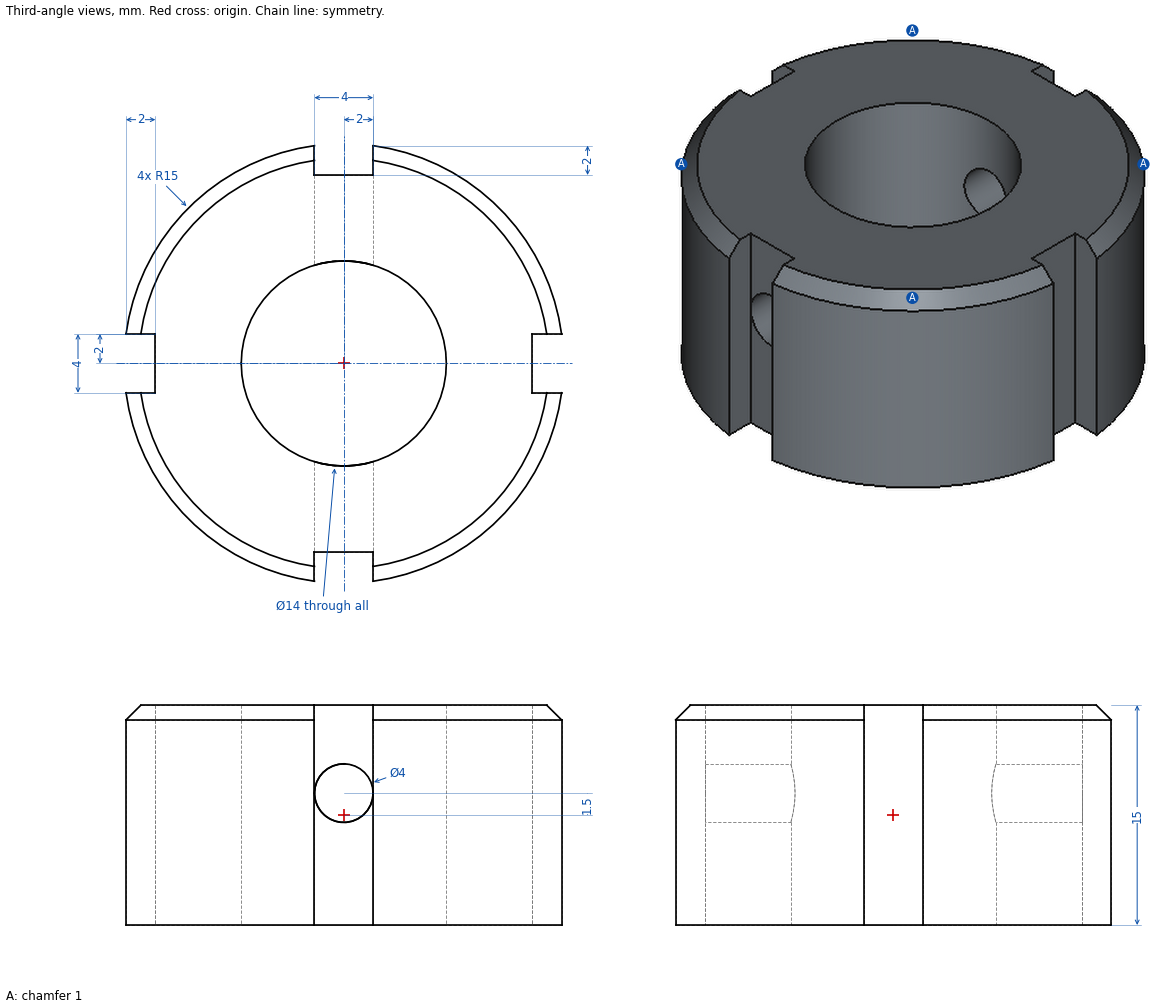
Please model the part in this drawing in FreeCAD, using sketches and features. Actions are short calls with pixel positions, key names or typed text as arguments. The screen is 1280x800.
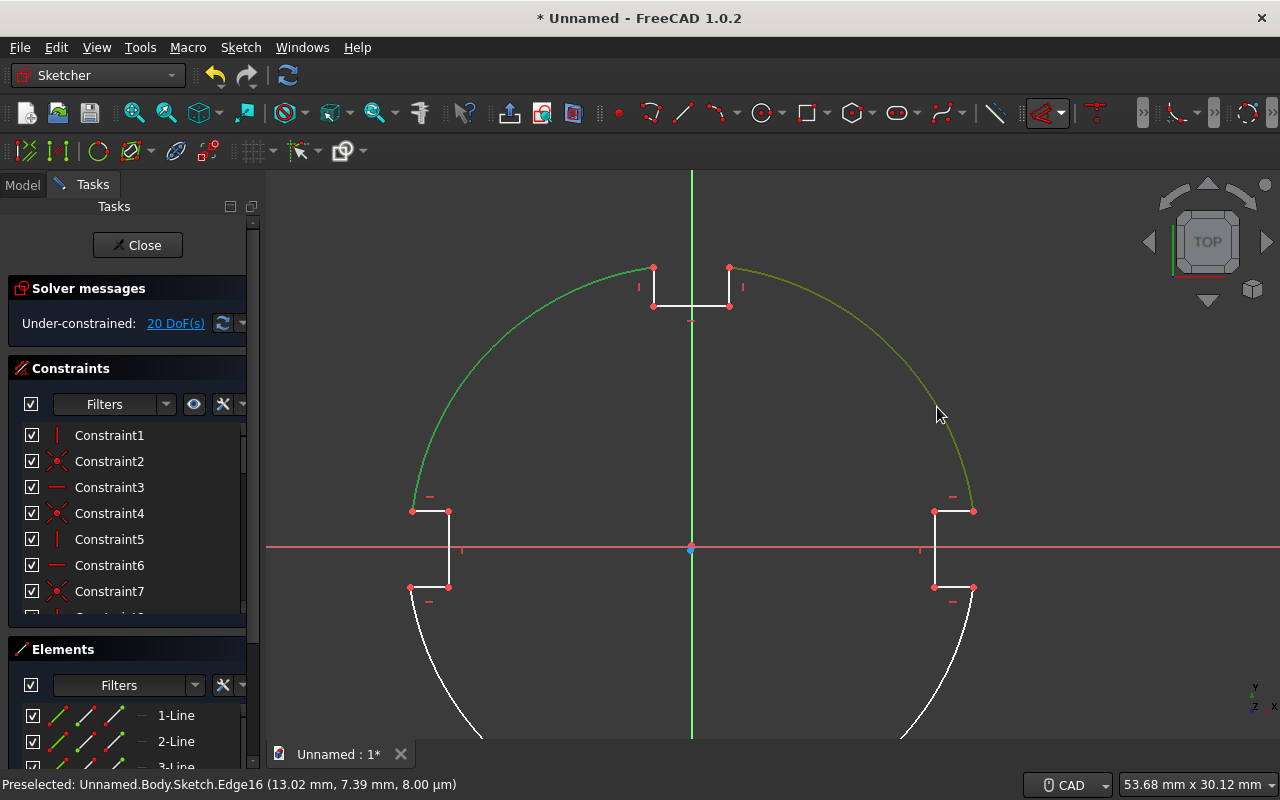
key(c)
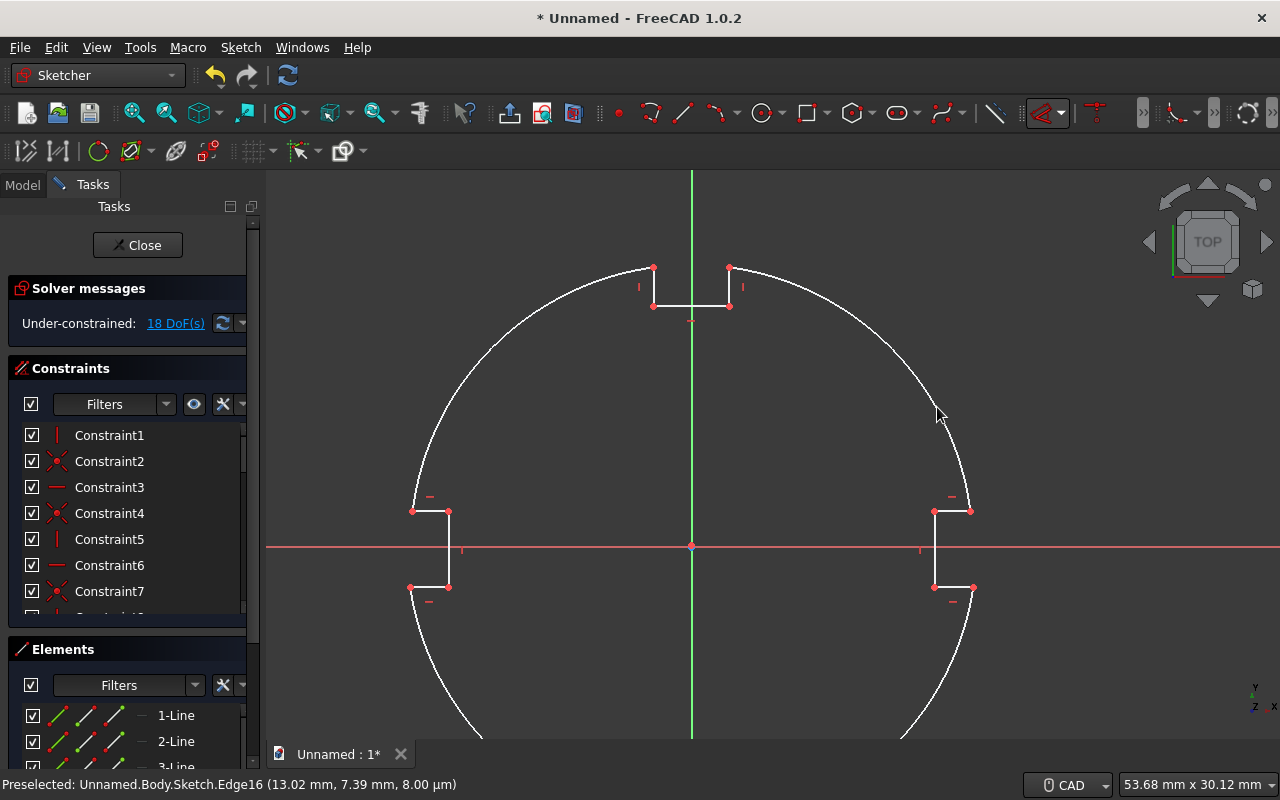
drag(682, 536, 702, 557)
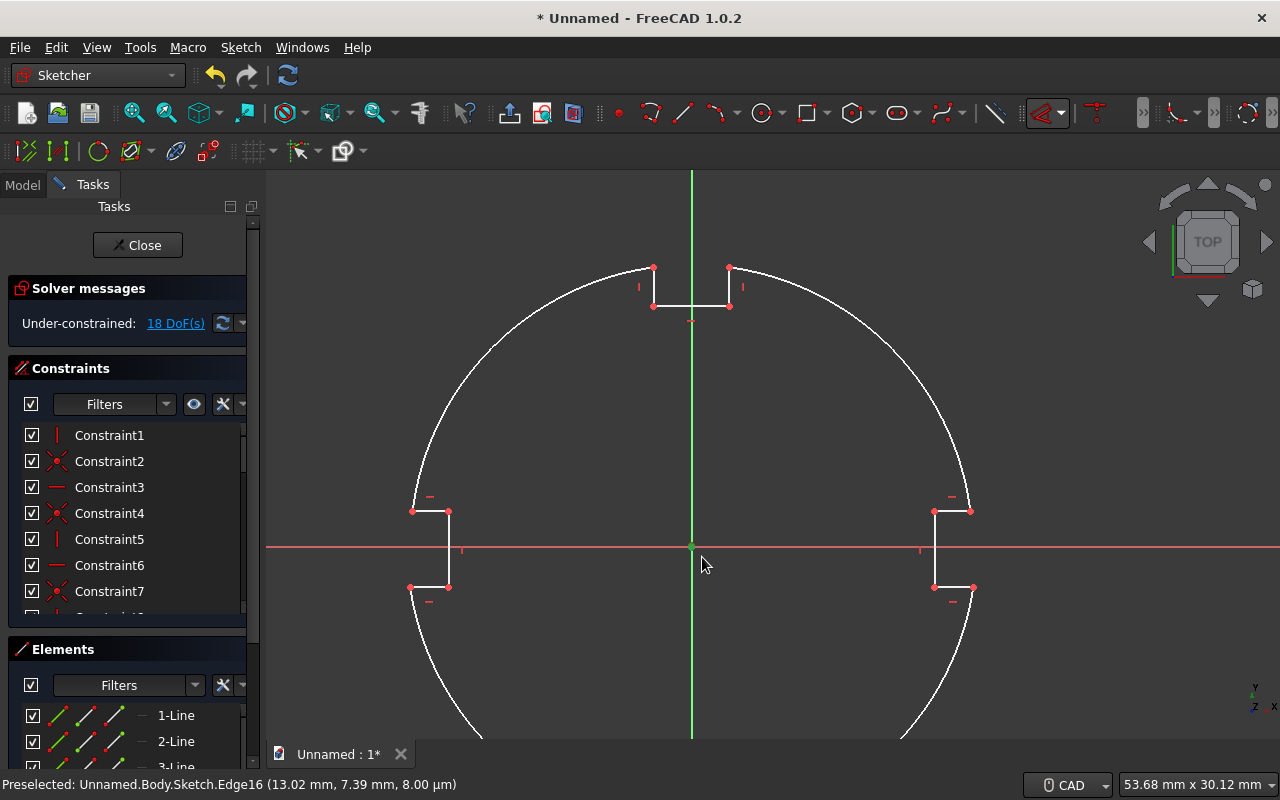
key(c)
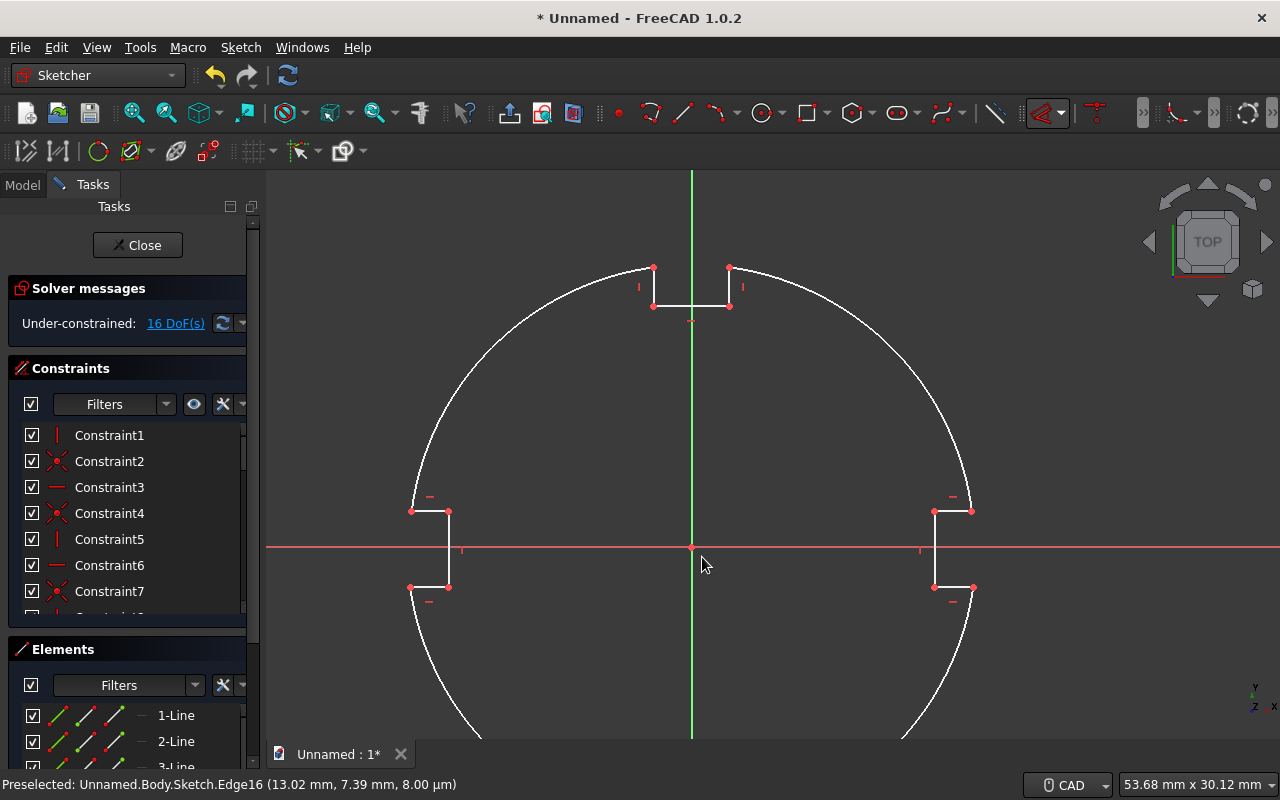
click(550, 303)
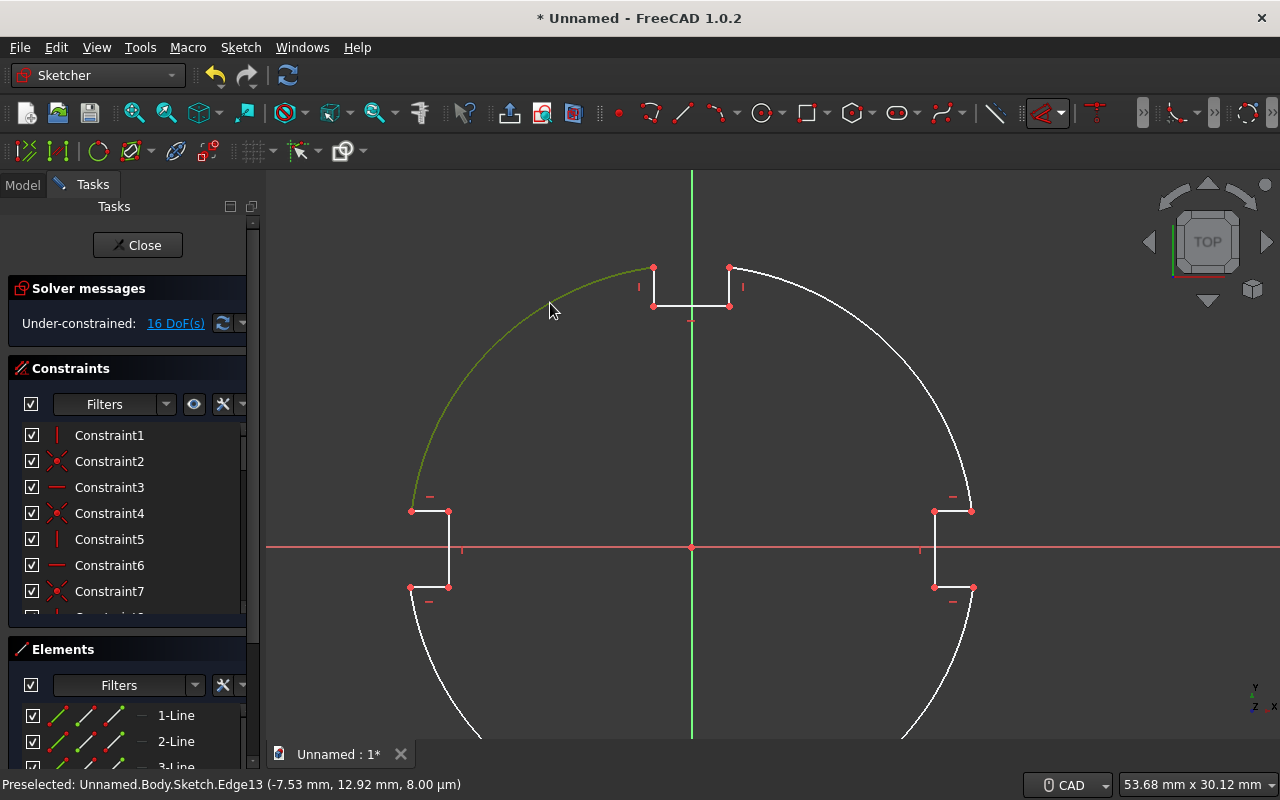
click(446, 691)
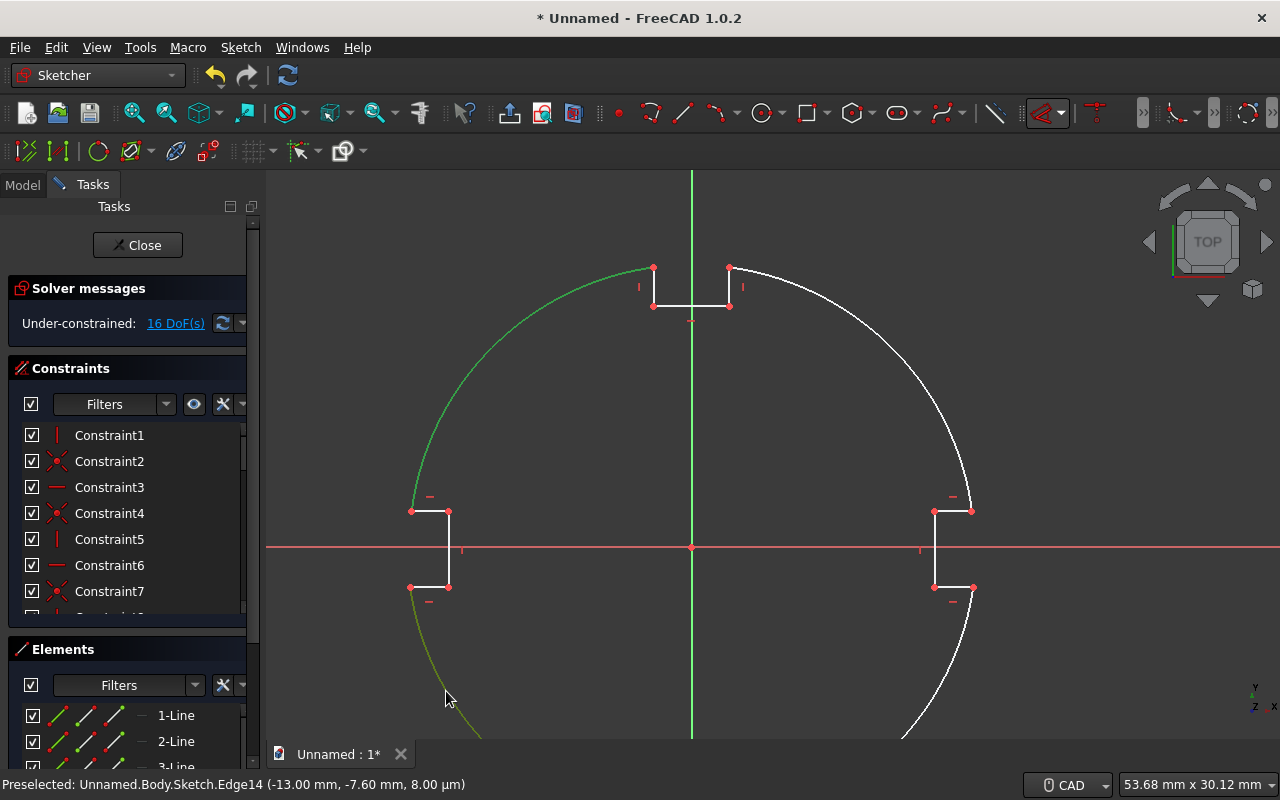
click(937, 691)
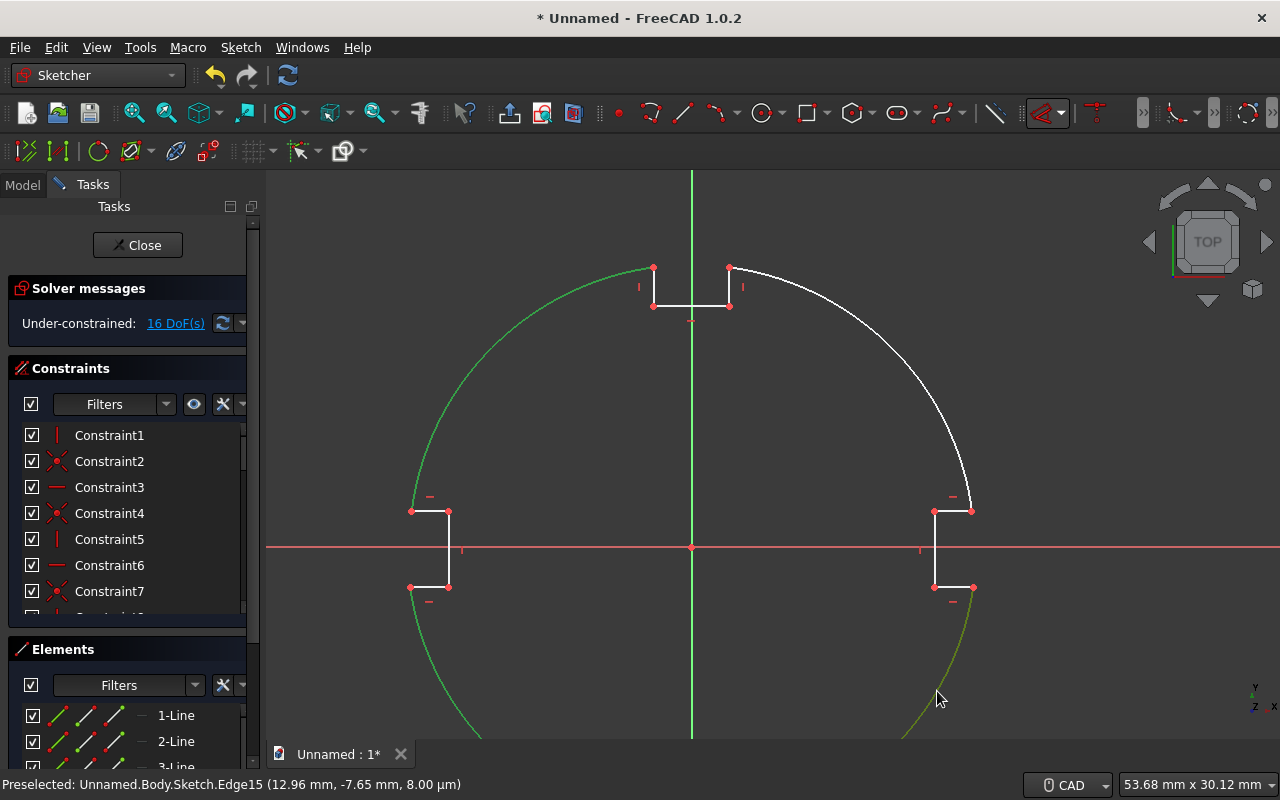
click(937, 407)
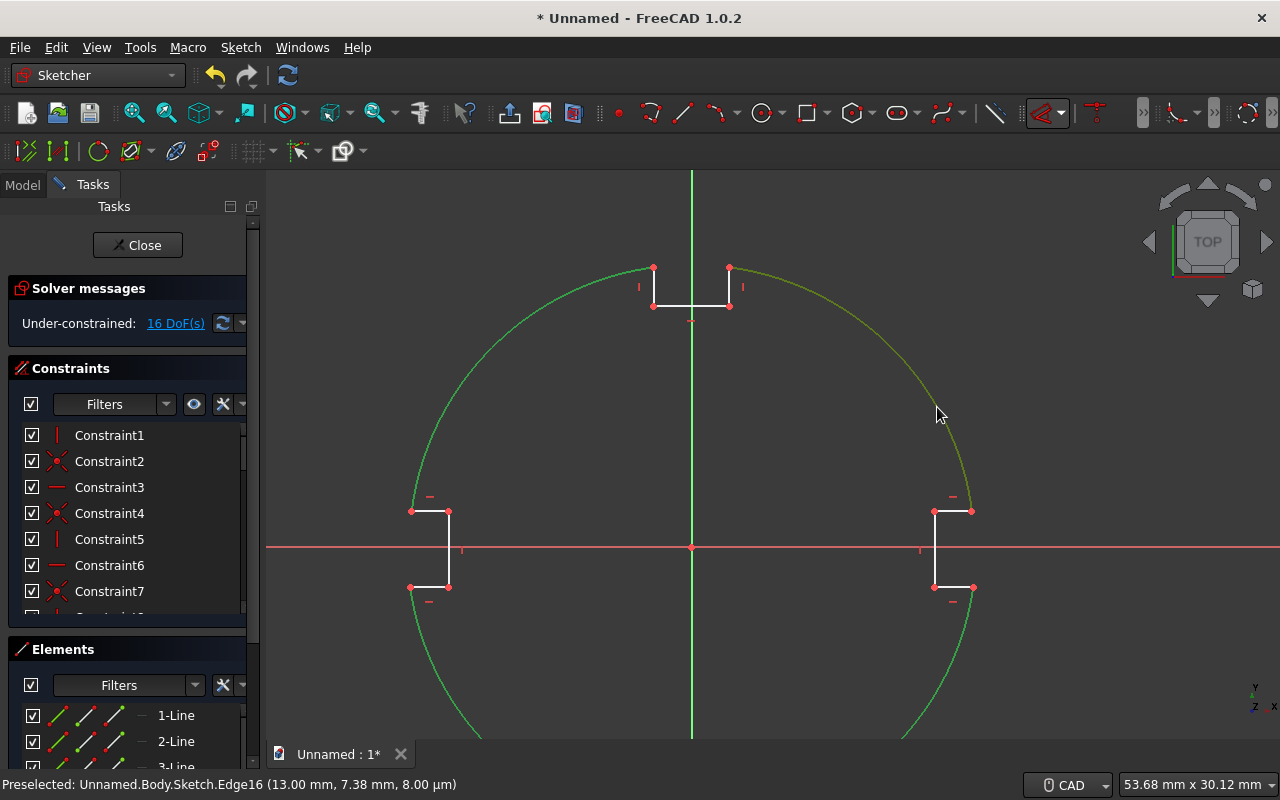
key(e)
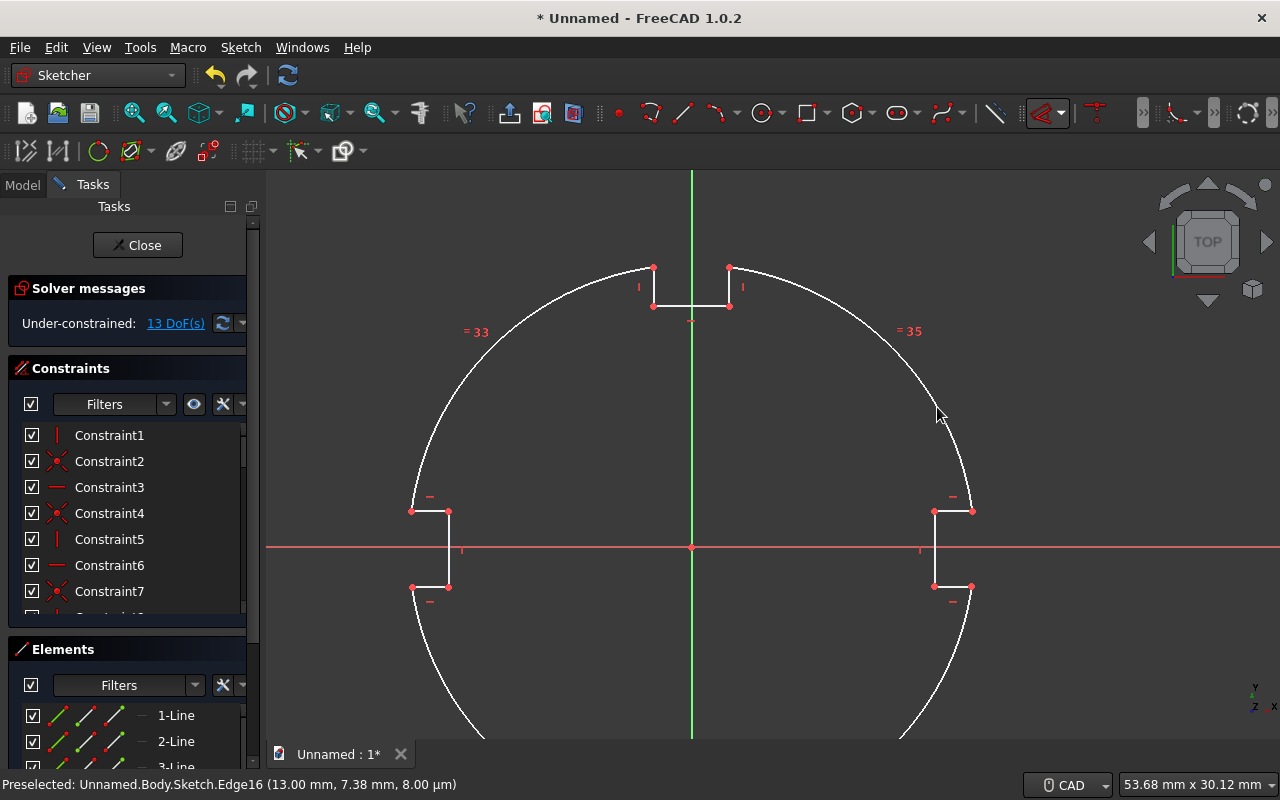
click(654, 306)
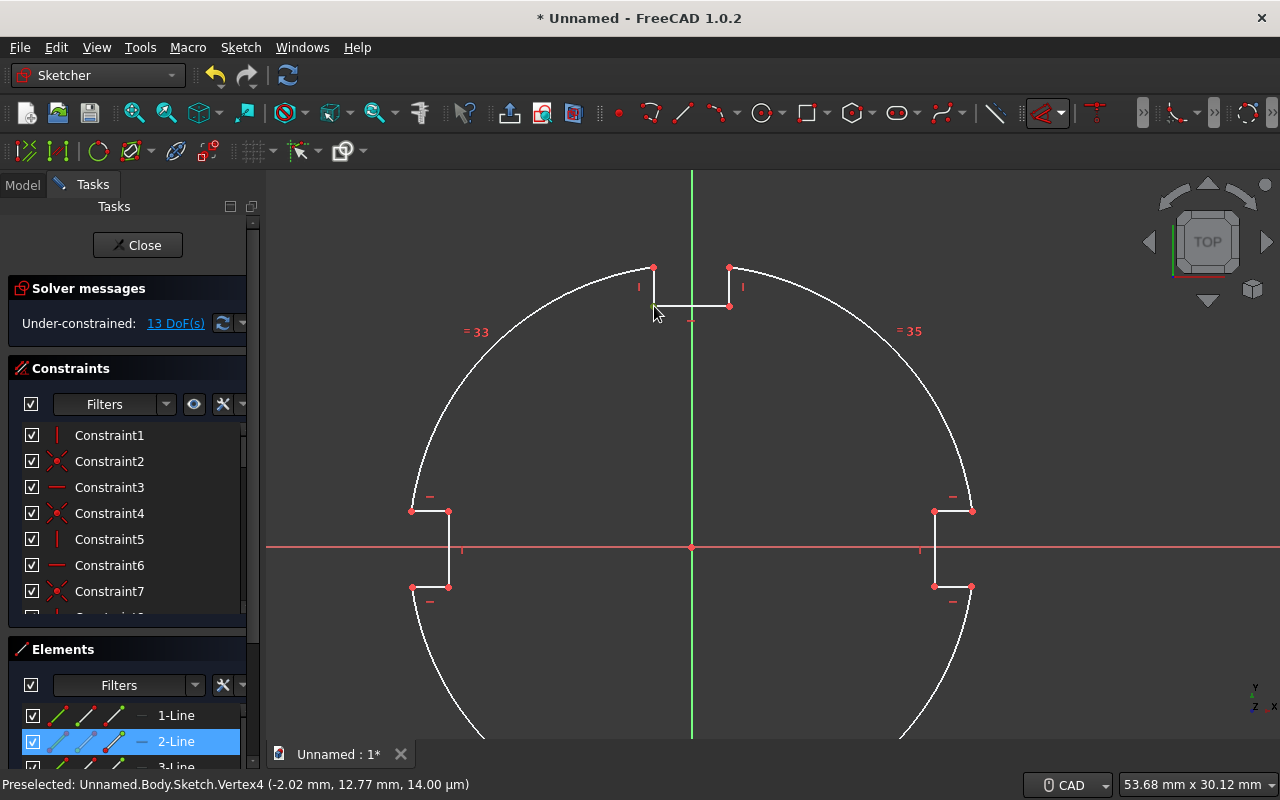
scroll(730, 266, down, 2)